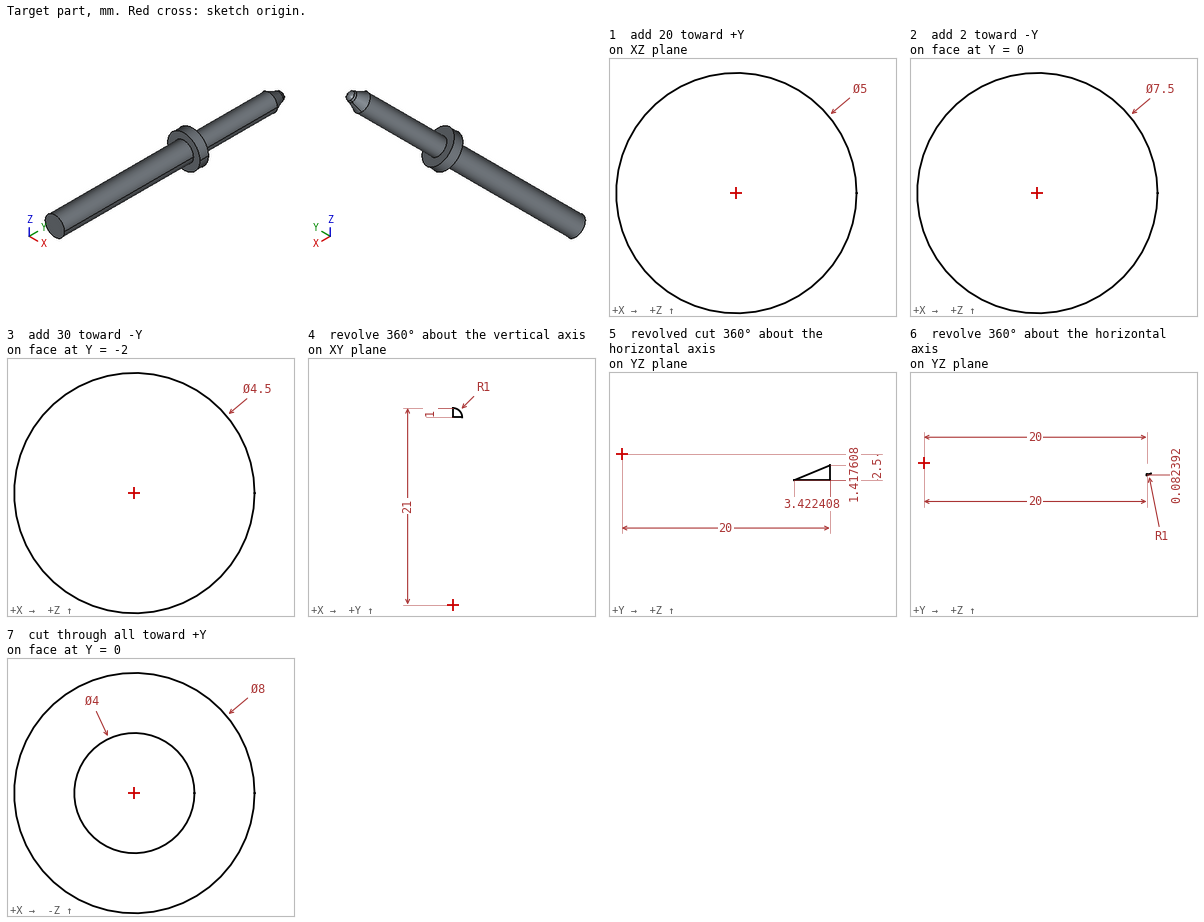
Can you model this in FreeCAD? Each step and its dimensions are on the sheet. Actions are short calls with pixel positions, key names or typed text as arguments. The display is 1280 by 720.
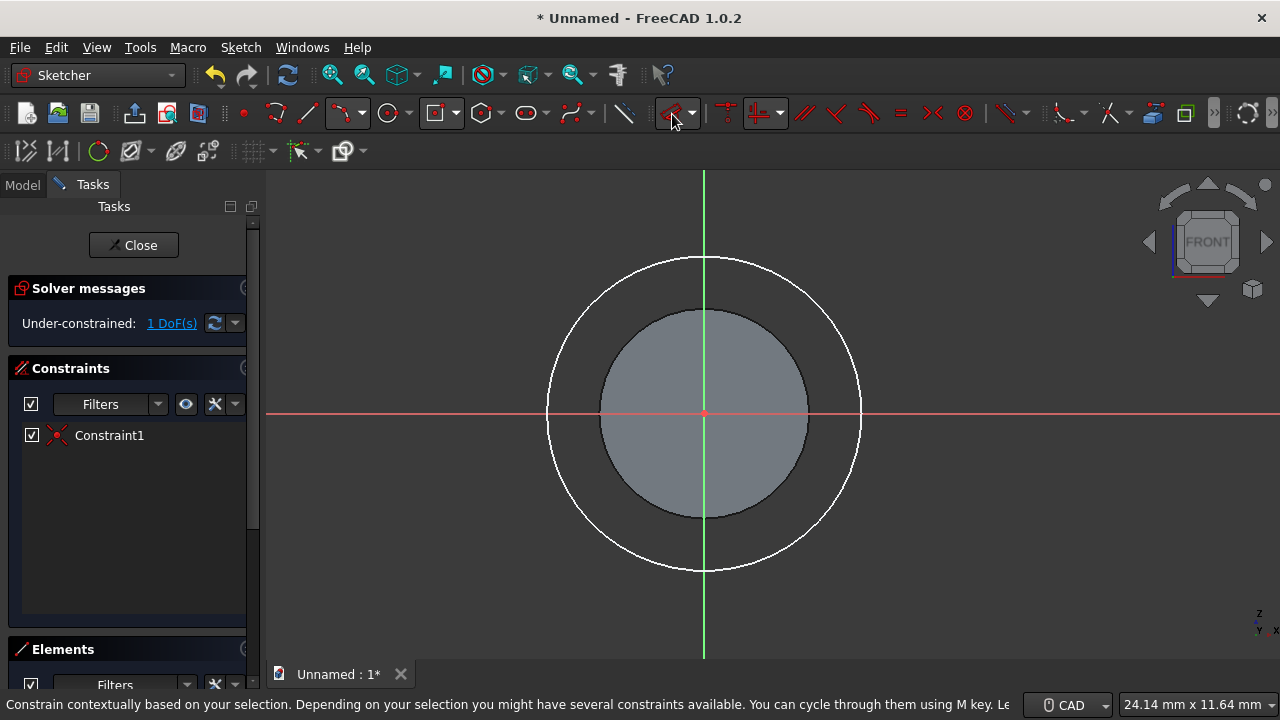
click(815, 302)
click(838, 279)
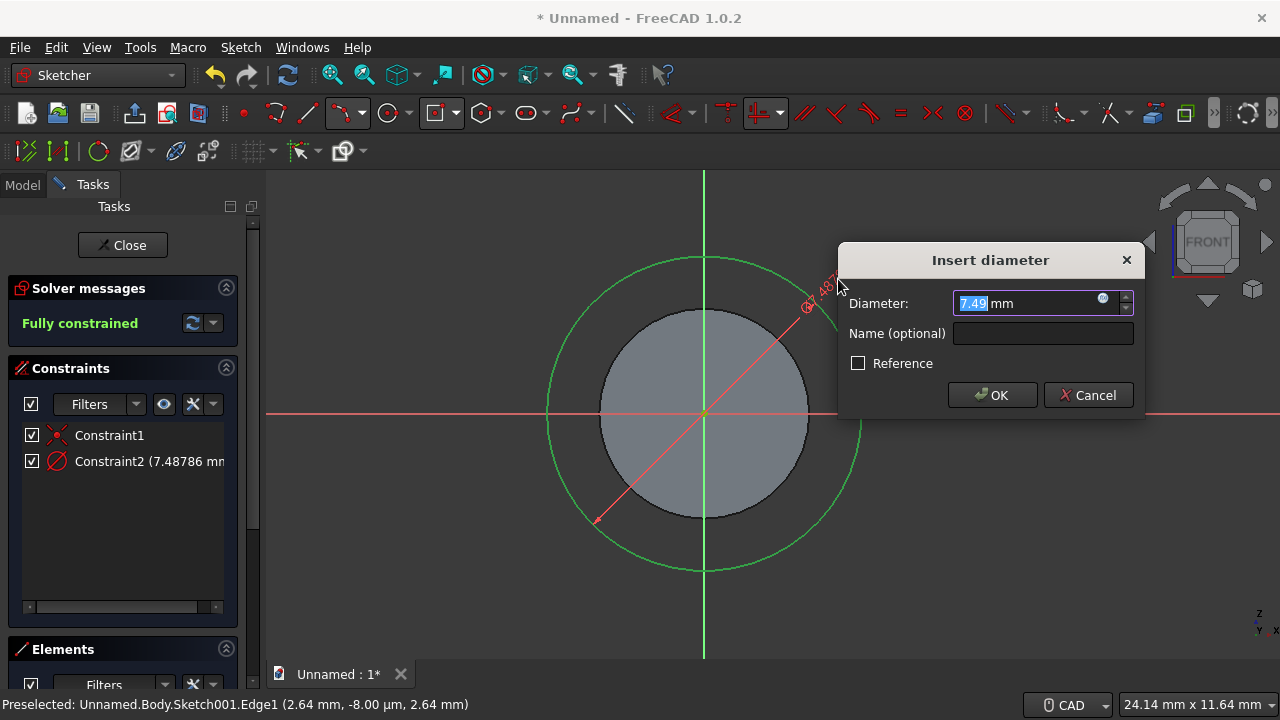
text(7.5)
key(Return)
key(Escape)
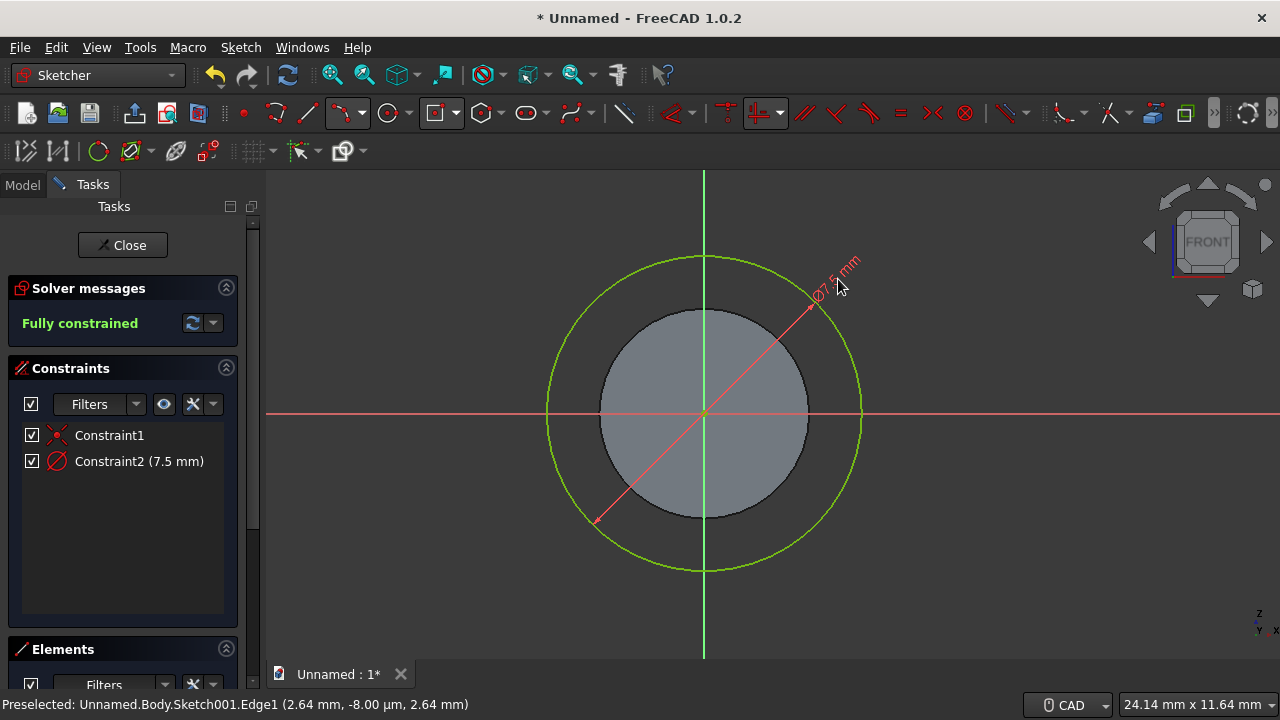
click(123, 245)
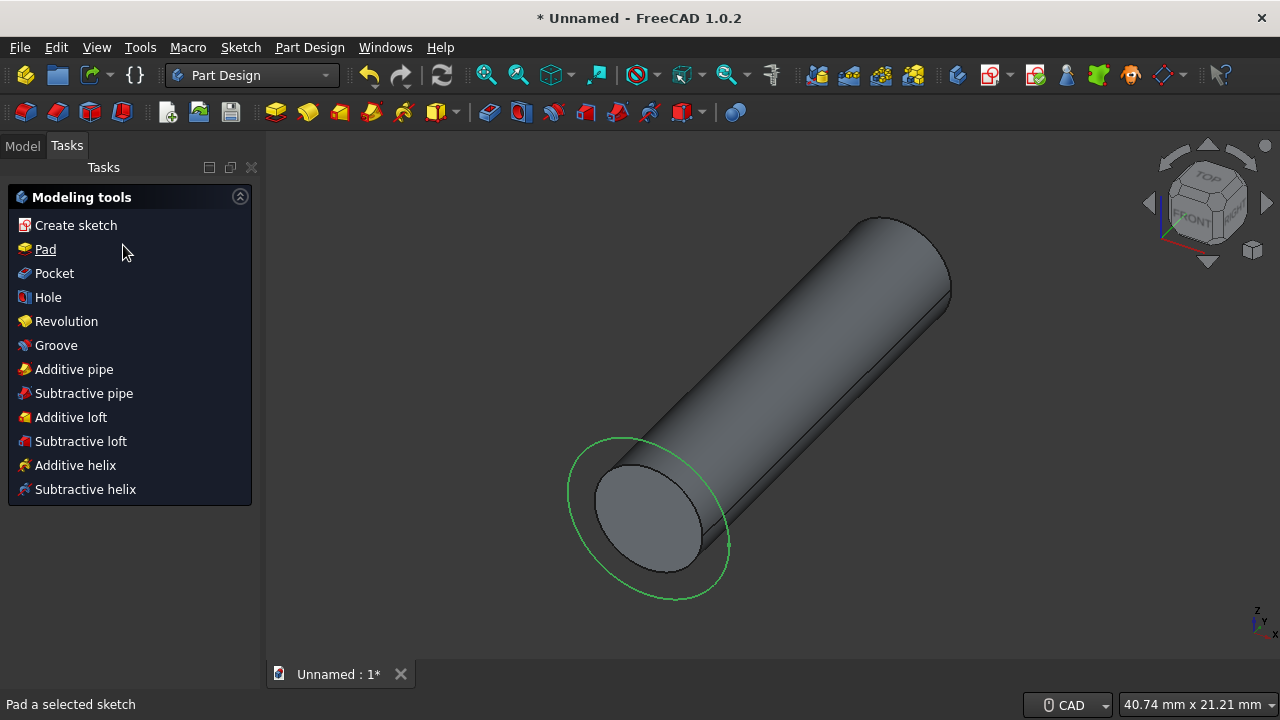
click(276, 112)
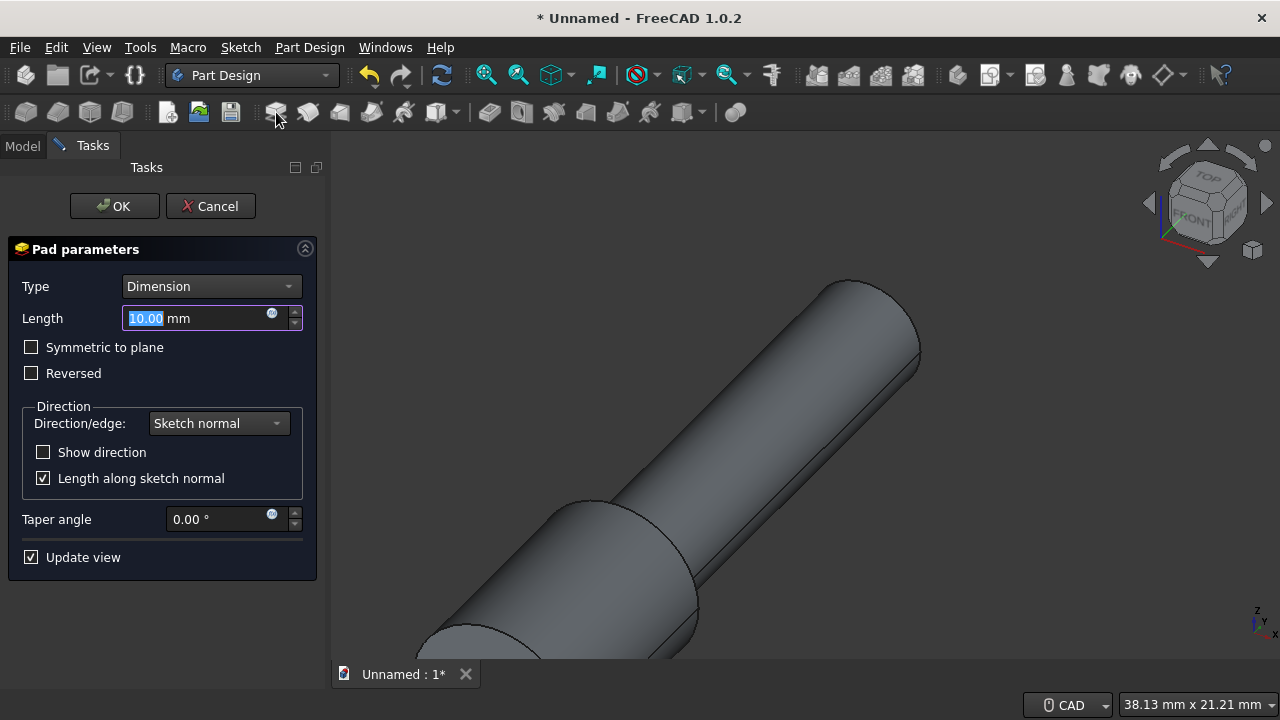
text(2)
key(Tab)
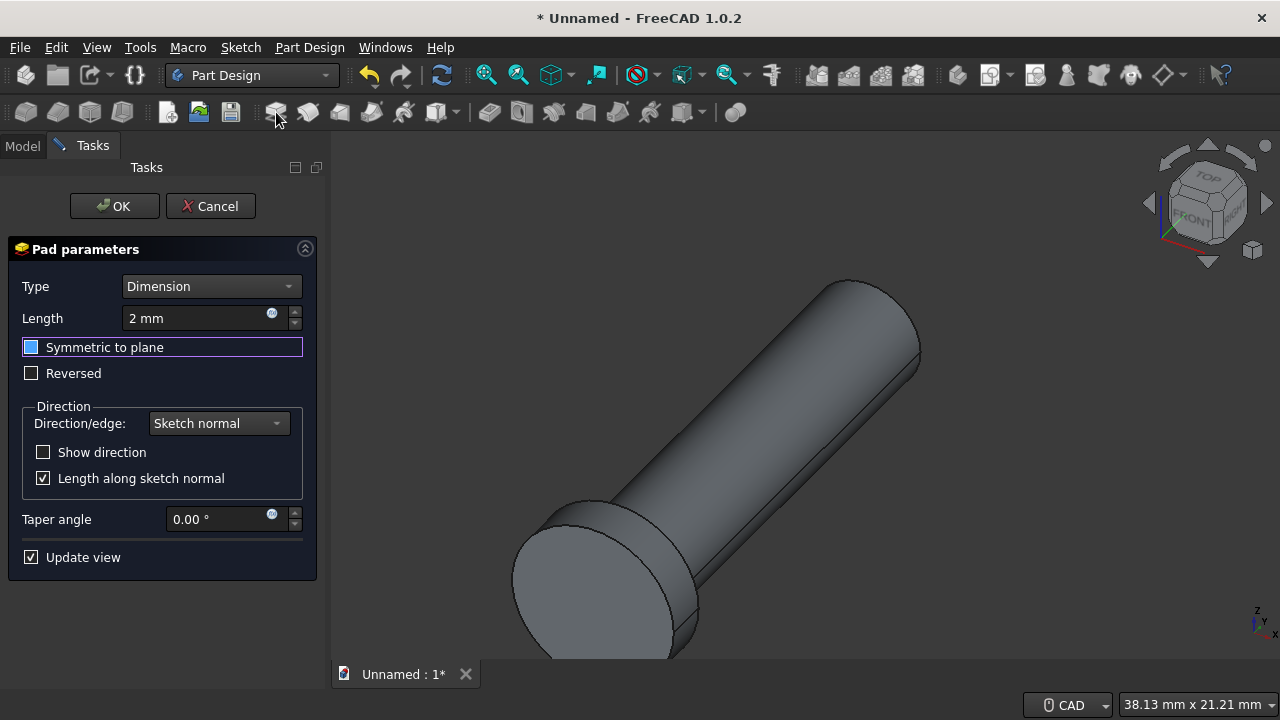
click(115, 206)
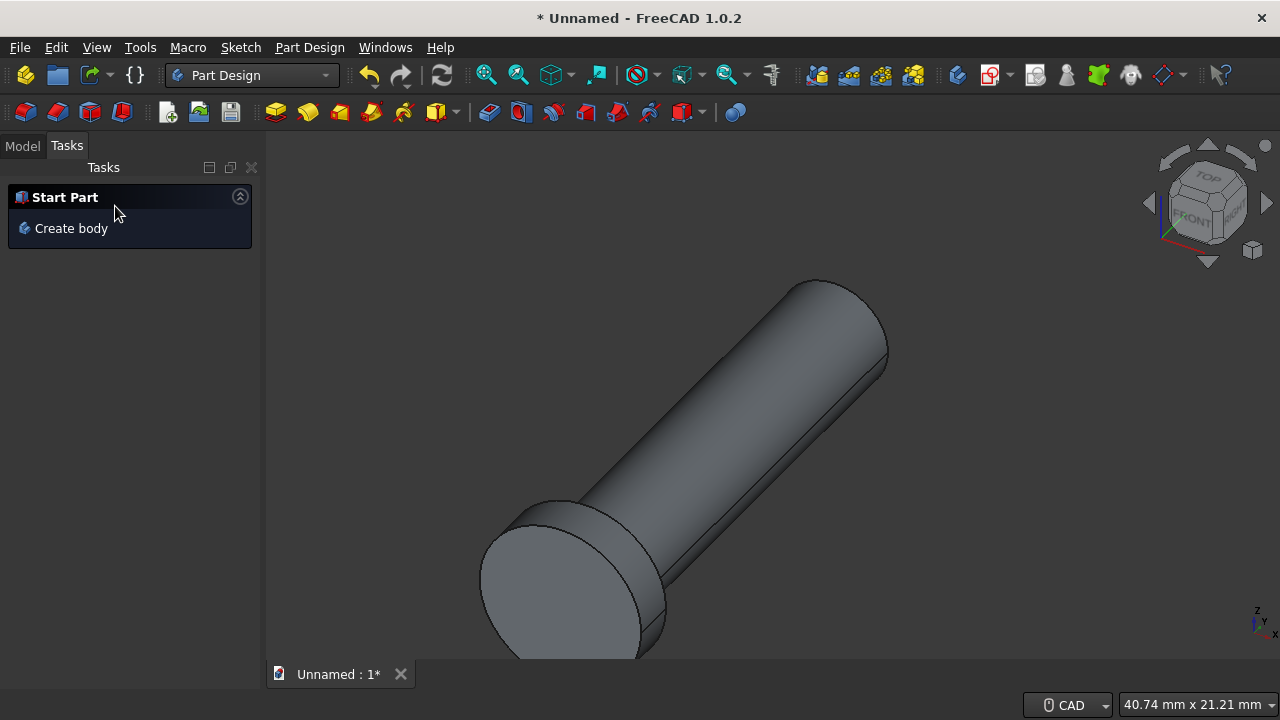
click(488, 76)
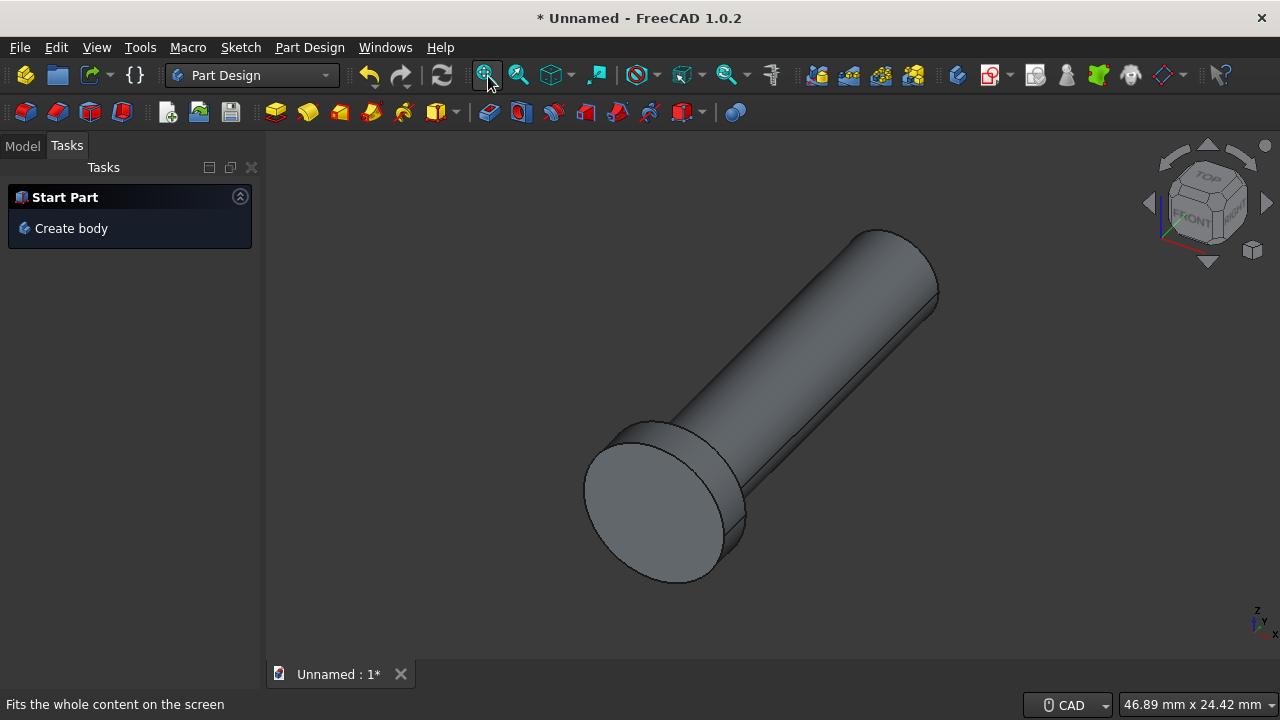
click(654, 512)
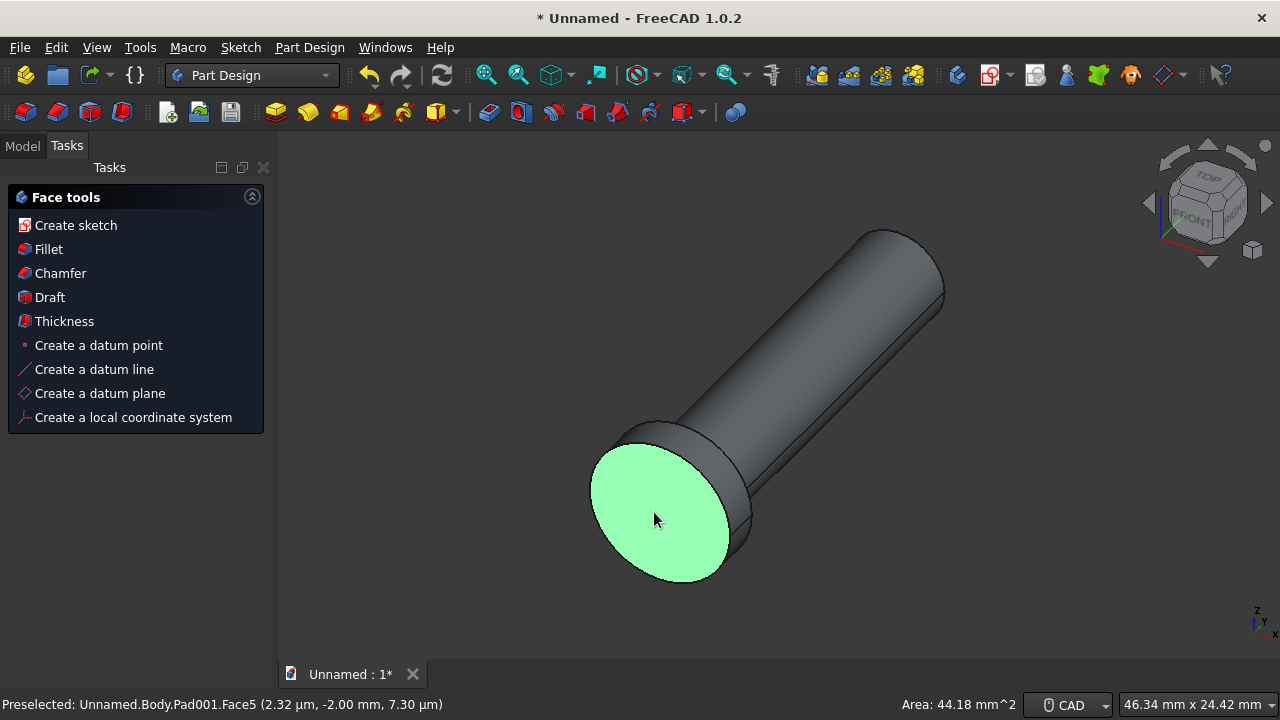
click(990, 76)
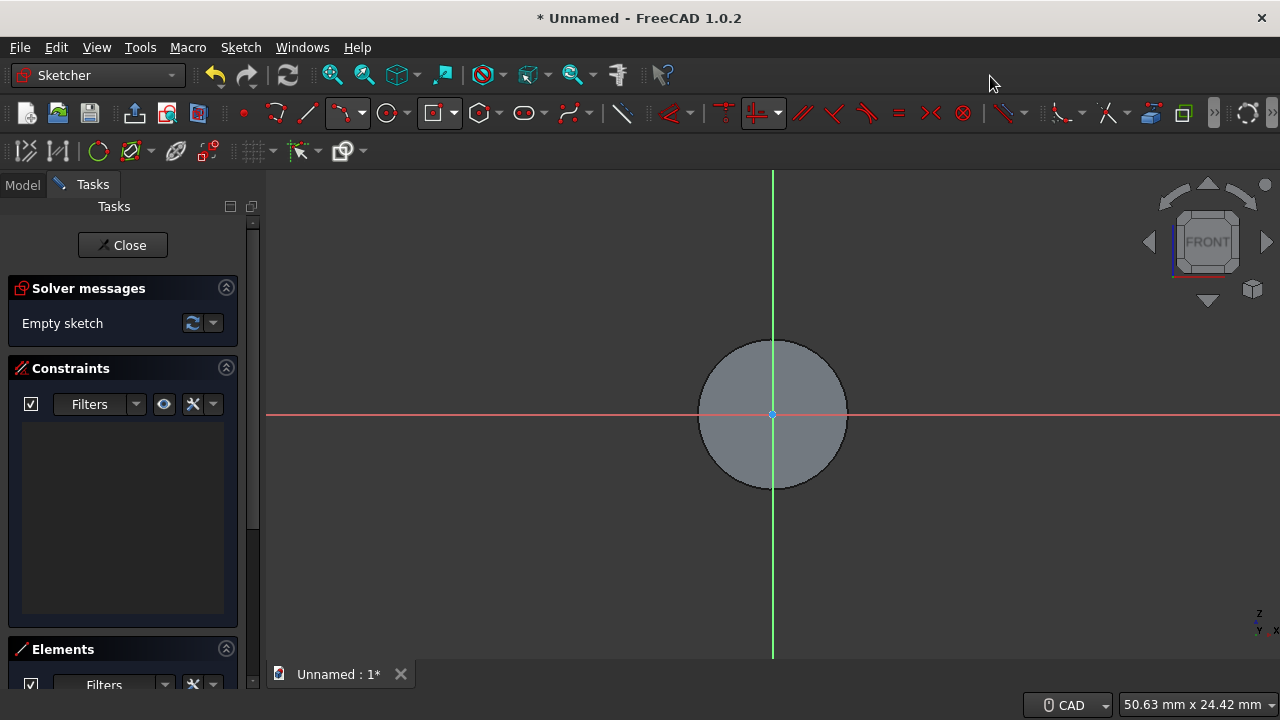
scroll(802, 415, up, 6)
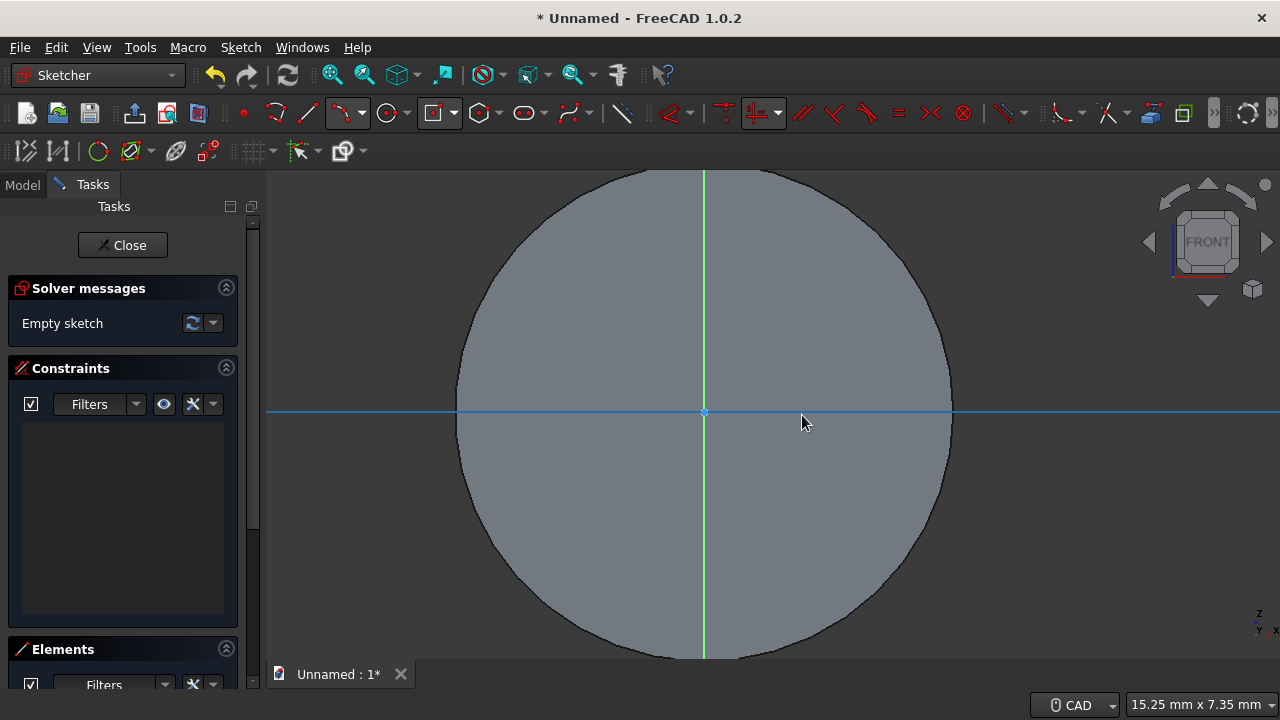
click(388, 114)